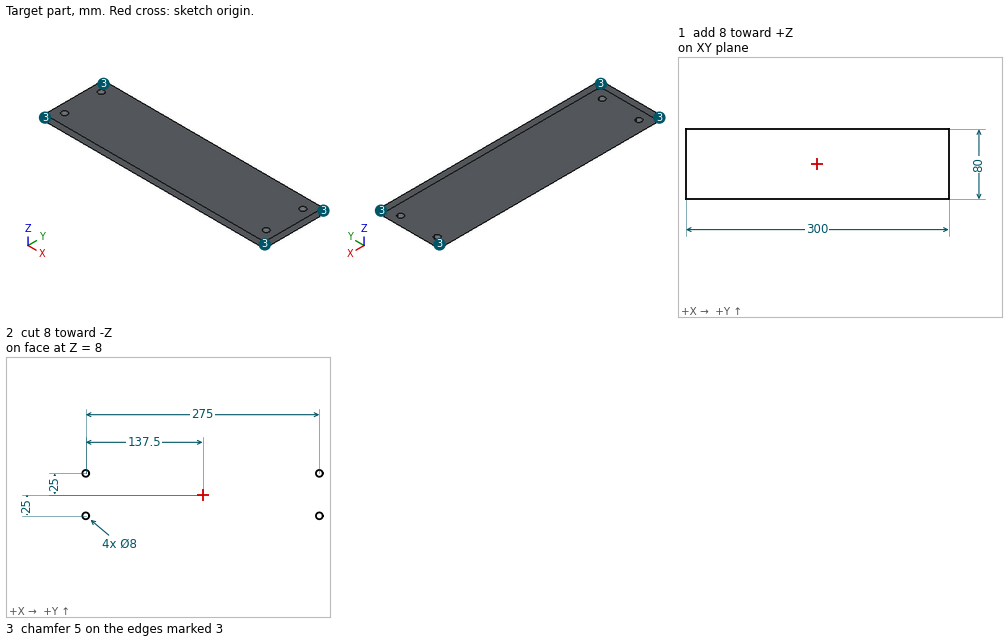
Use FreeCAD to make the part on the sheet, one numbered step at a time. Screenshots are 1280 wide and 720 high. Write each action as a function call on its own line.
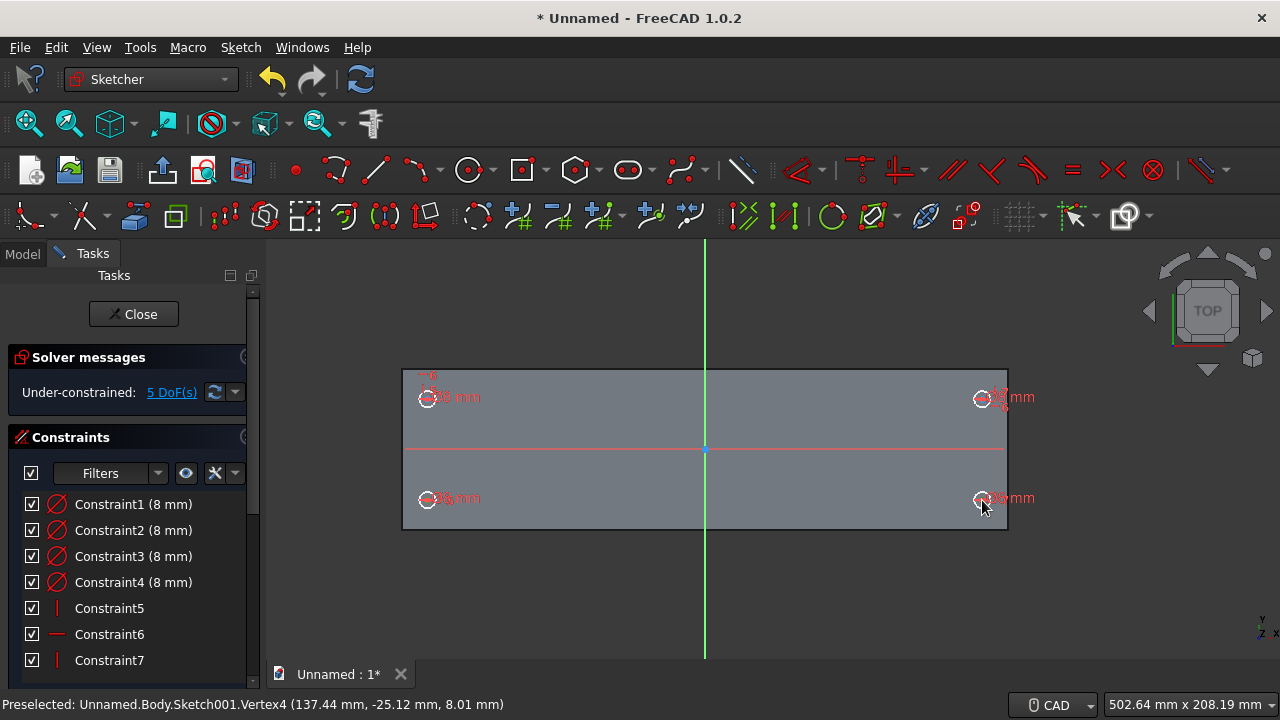
key(h)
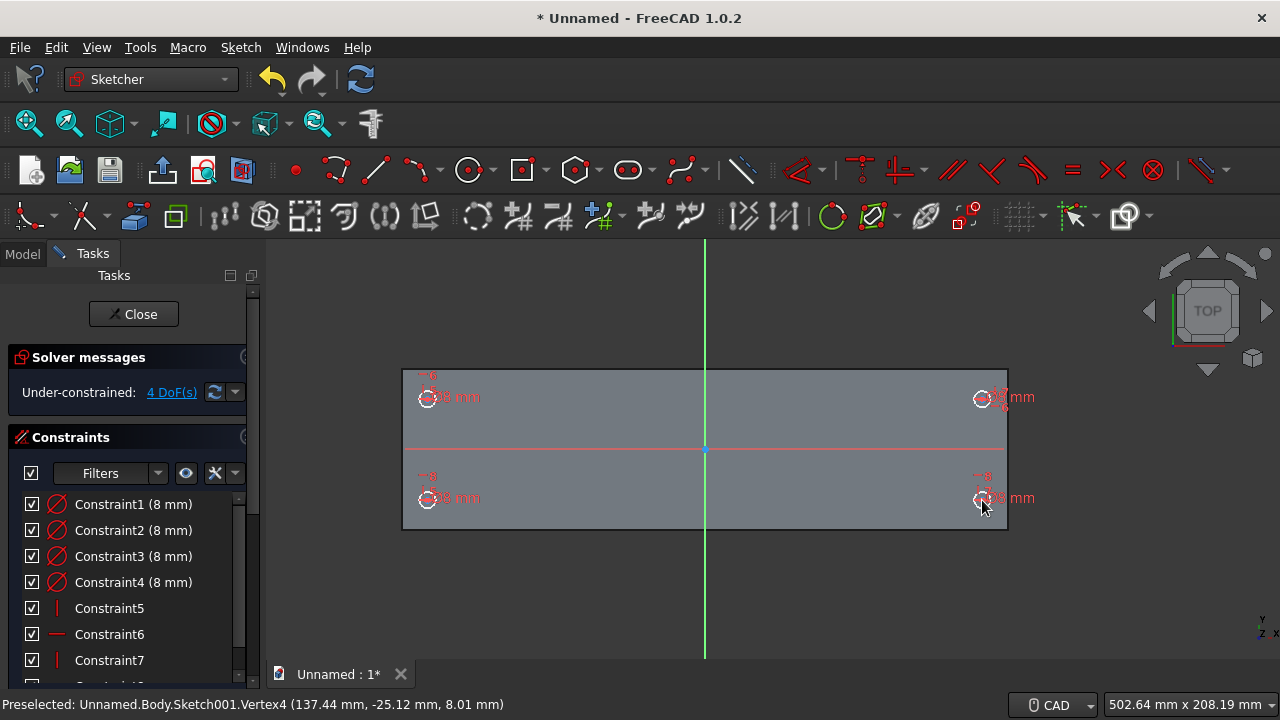
key(d)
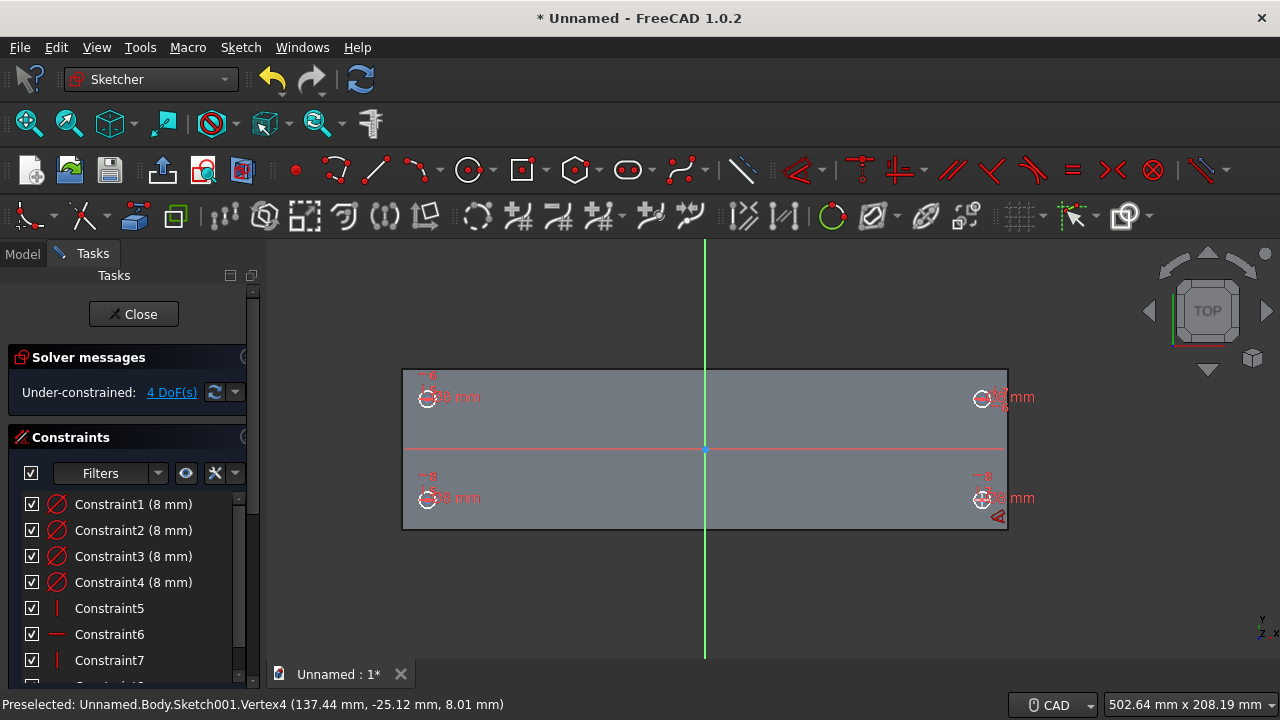
click(428, 399)
click(394, 424)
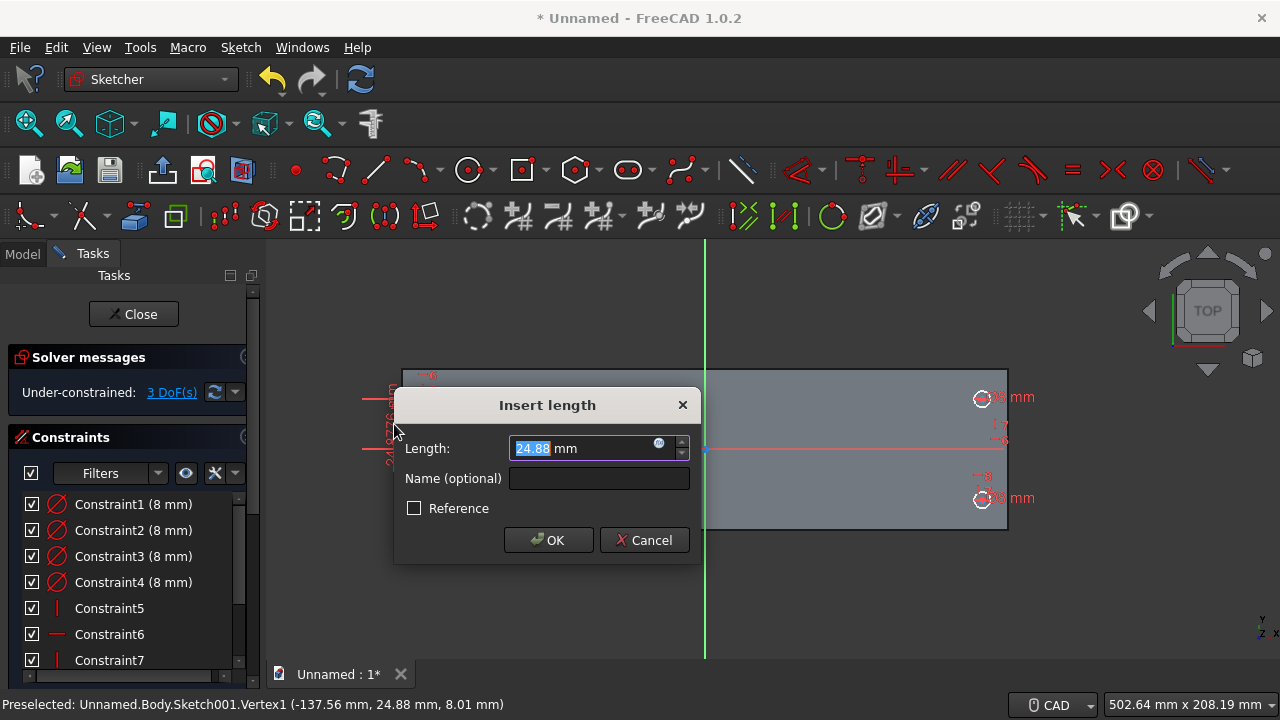
text(25)
key(Return)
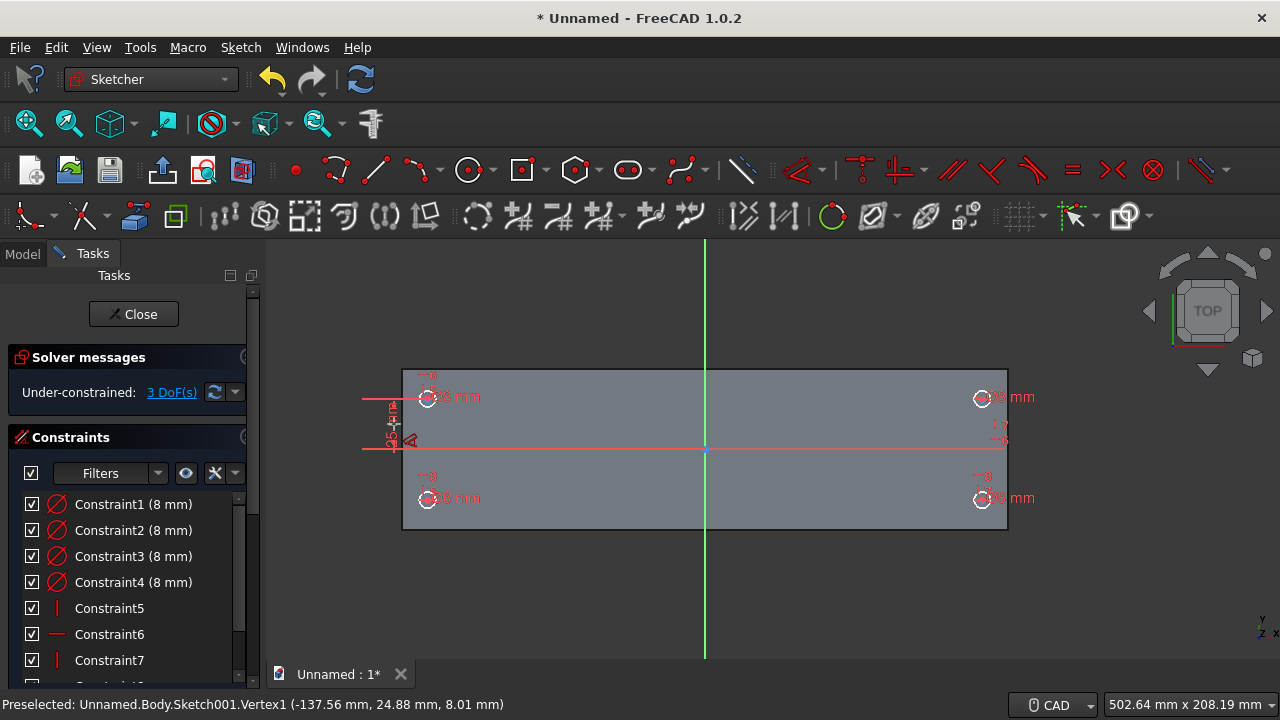
click(428, 500)
click(394, 475)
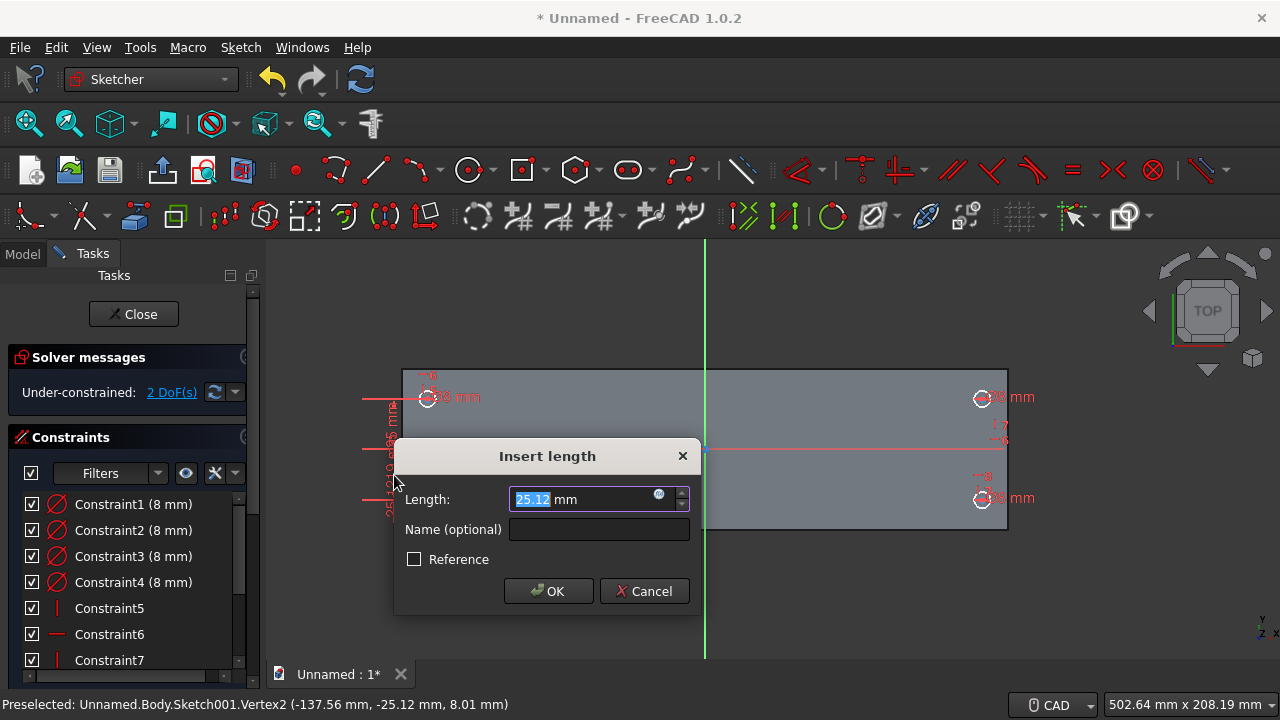
text(25)
key(Return)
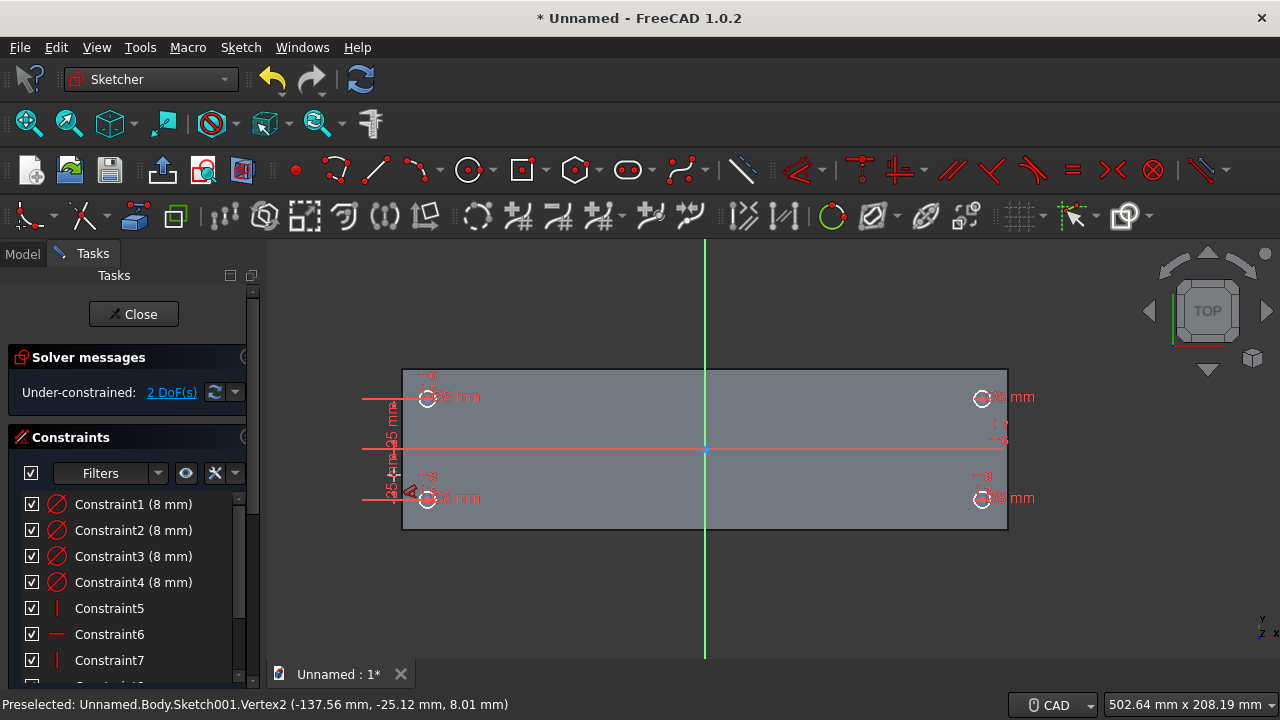
click(428, 399)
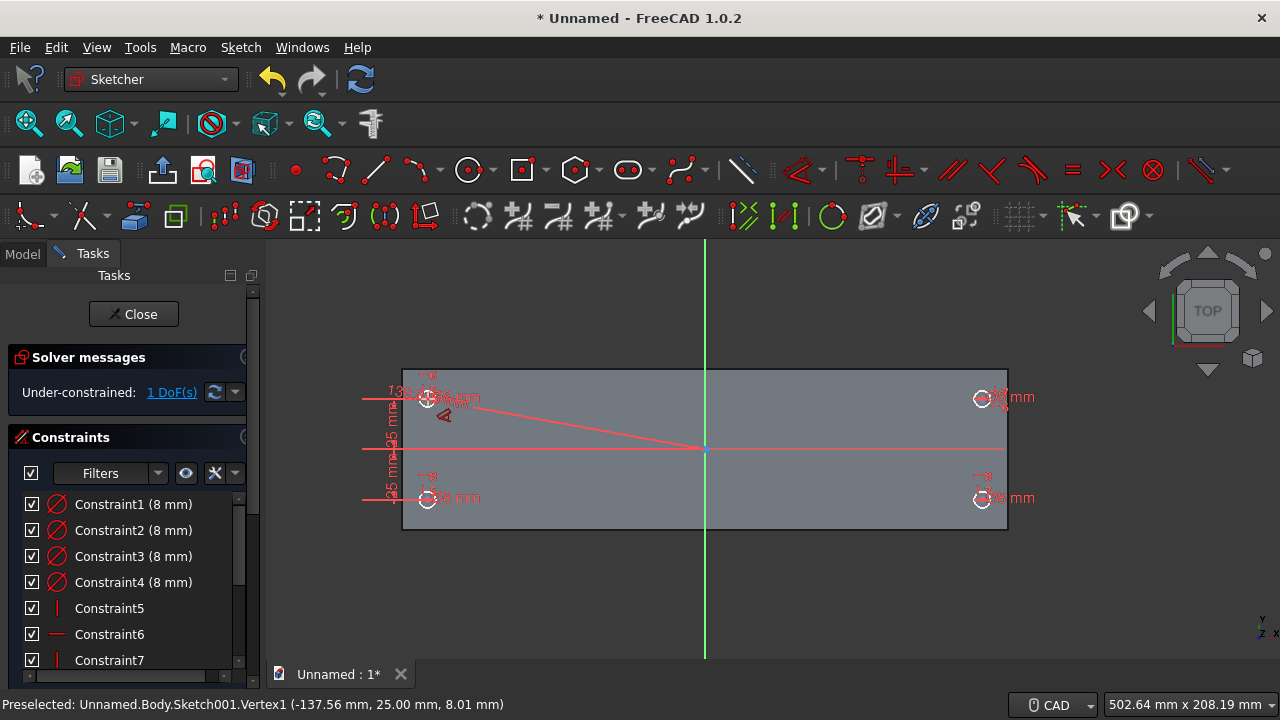
click(982, 399)
click(577, 365)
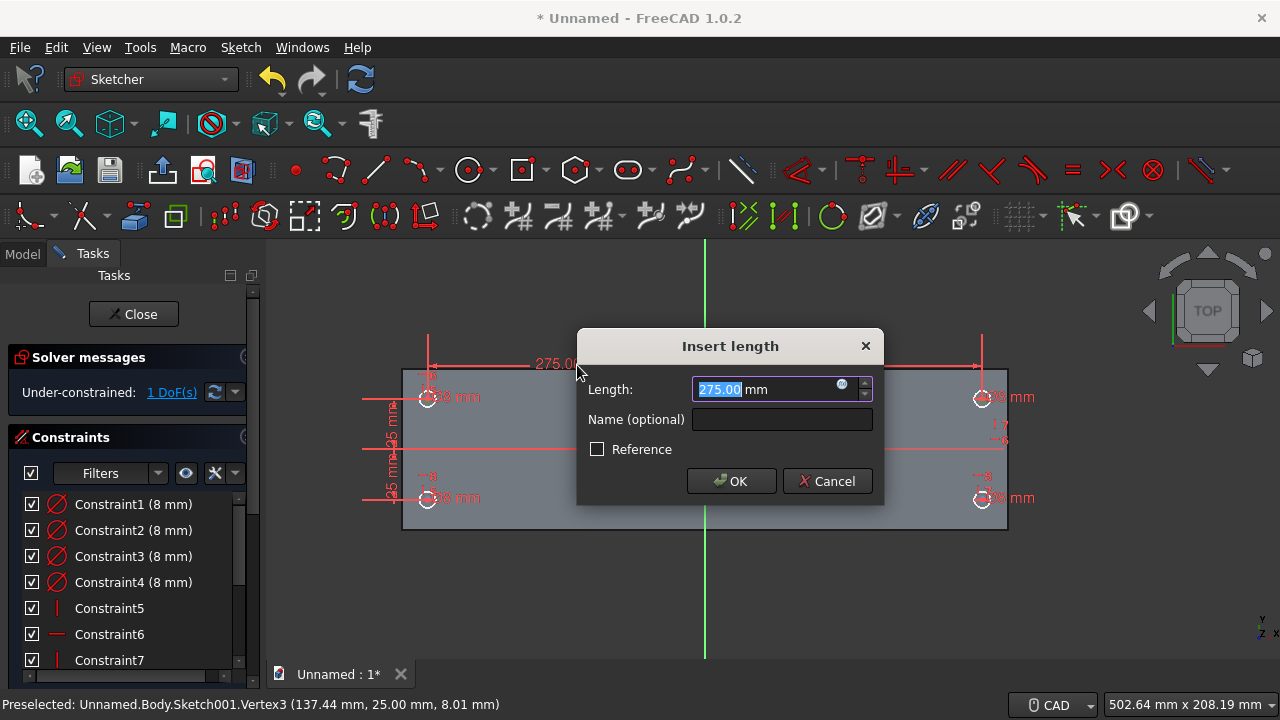
text(275)
key(Return)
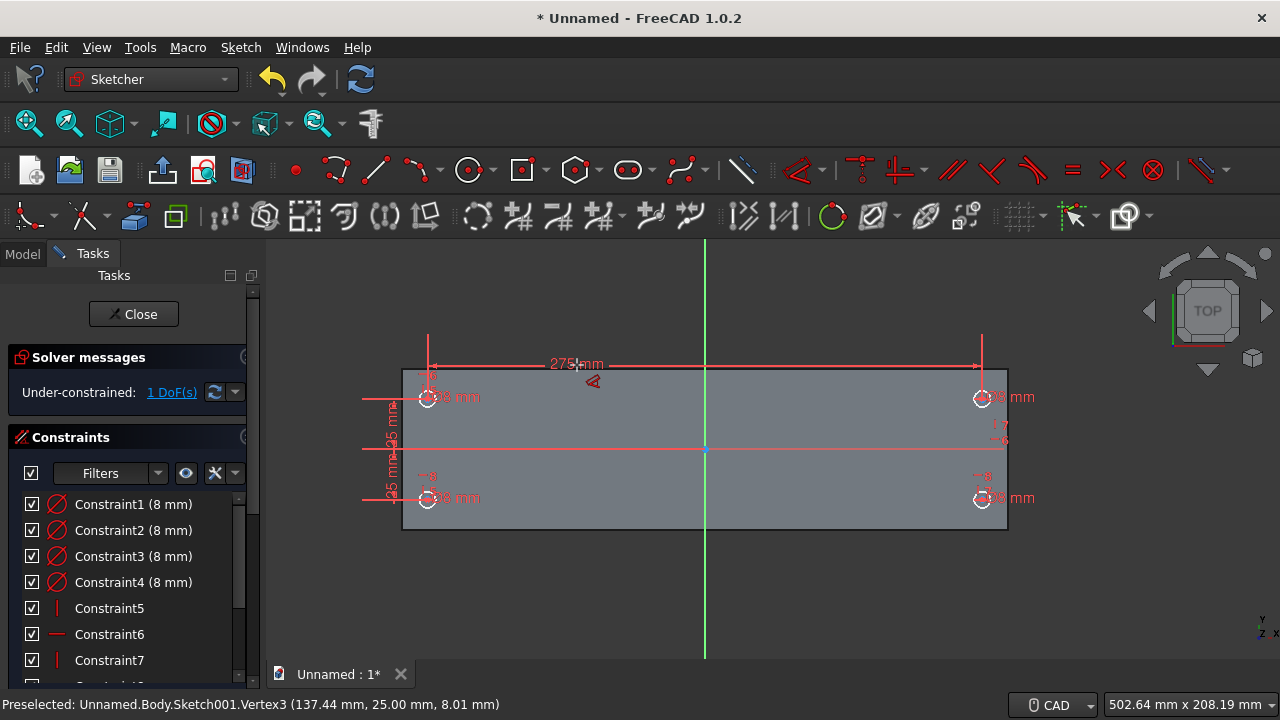
click(428, 399)
click(502, 365)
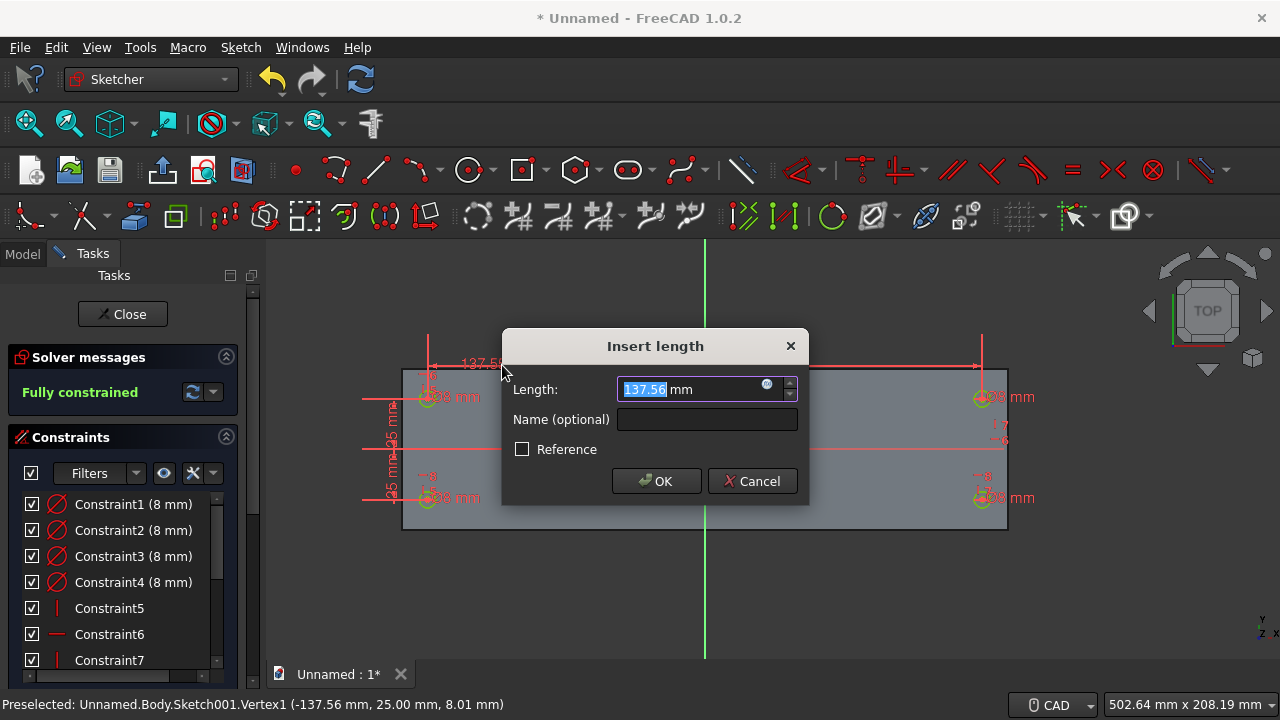
text(137.5)
key(Return)
key(Escape)